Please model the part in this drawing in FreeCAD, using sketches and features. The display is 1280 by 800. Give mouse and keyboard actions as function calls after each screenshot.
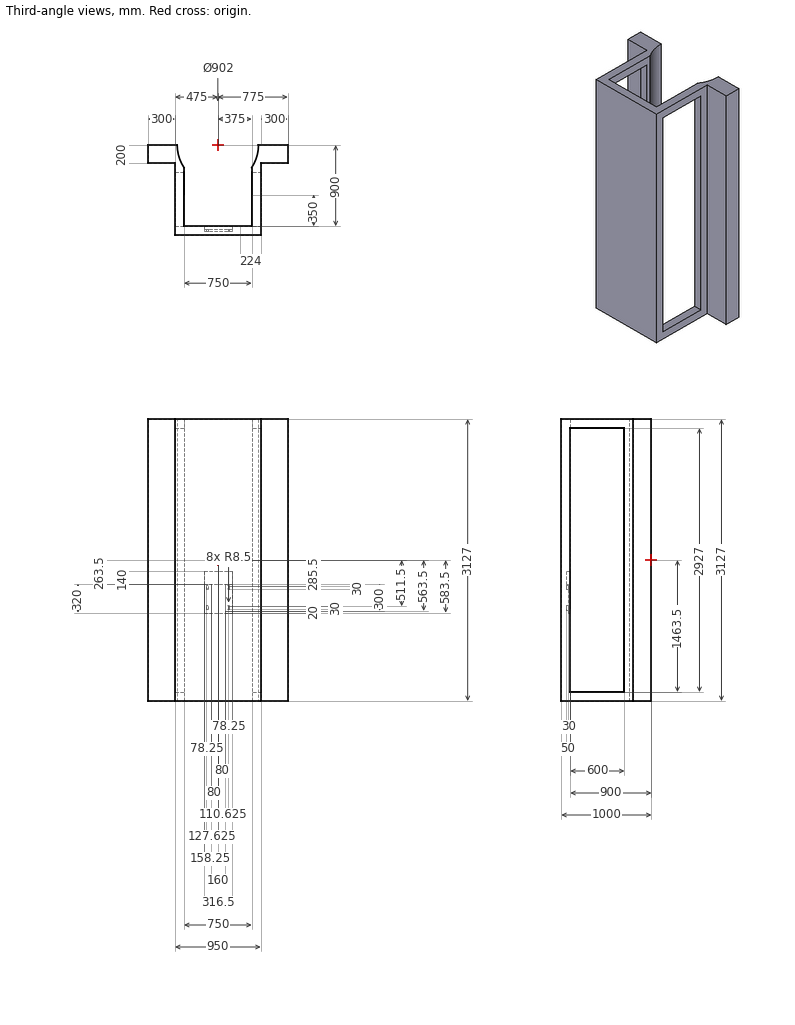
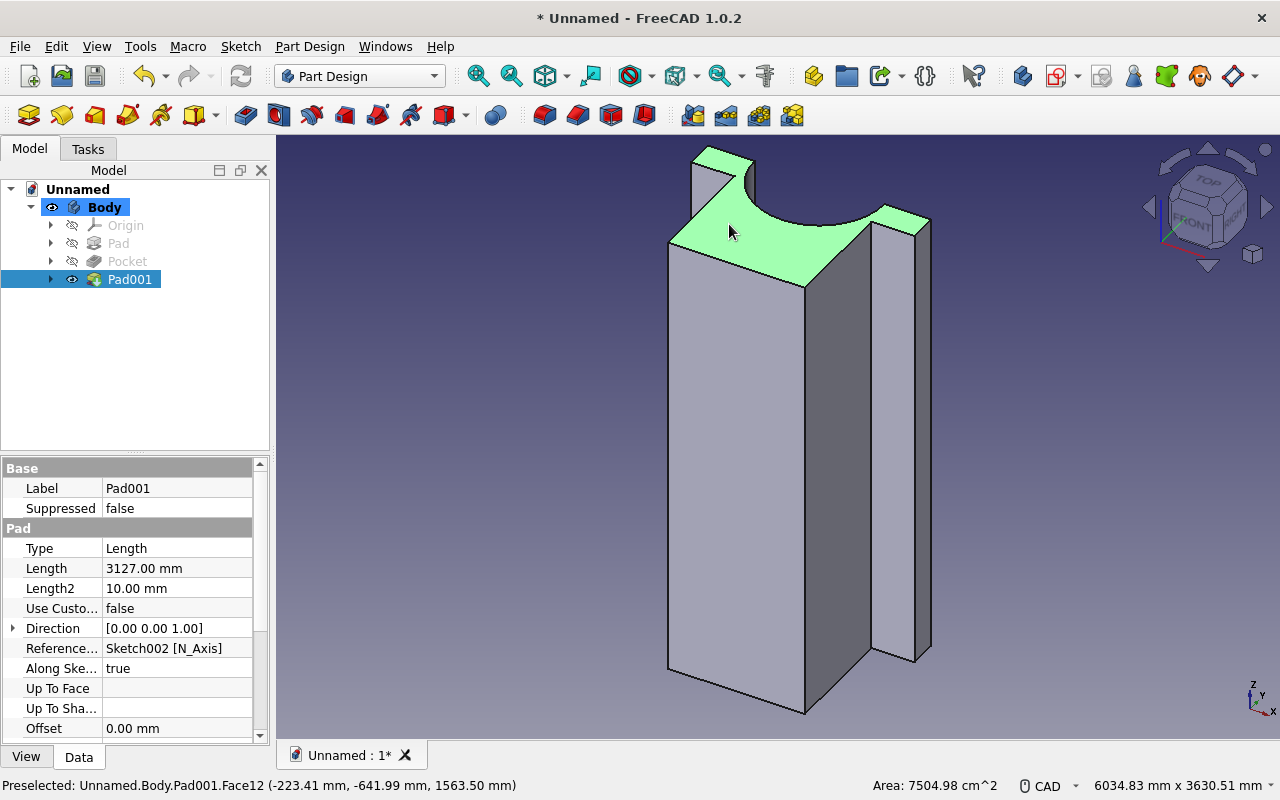
click(1056, 76)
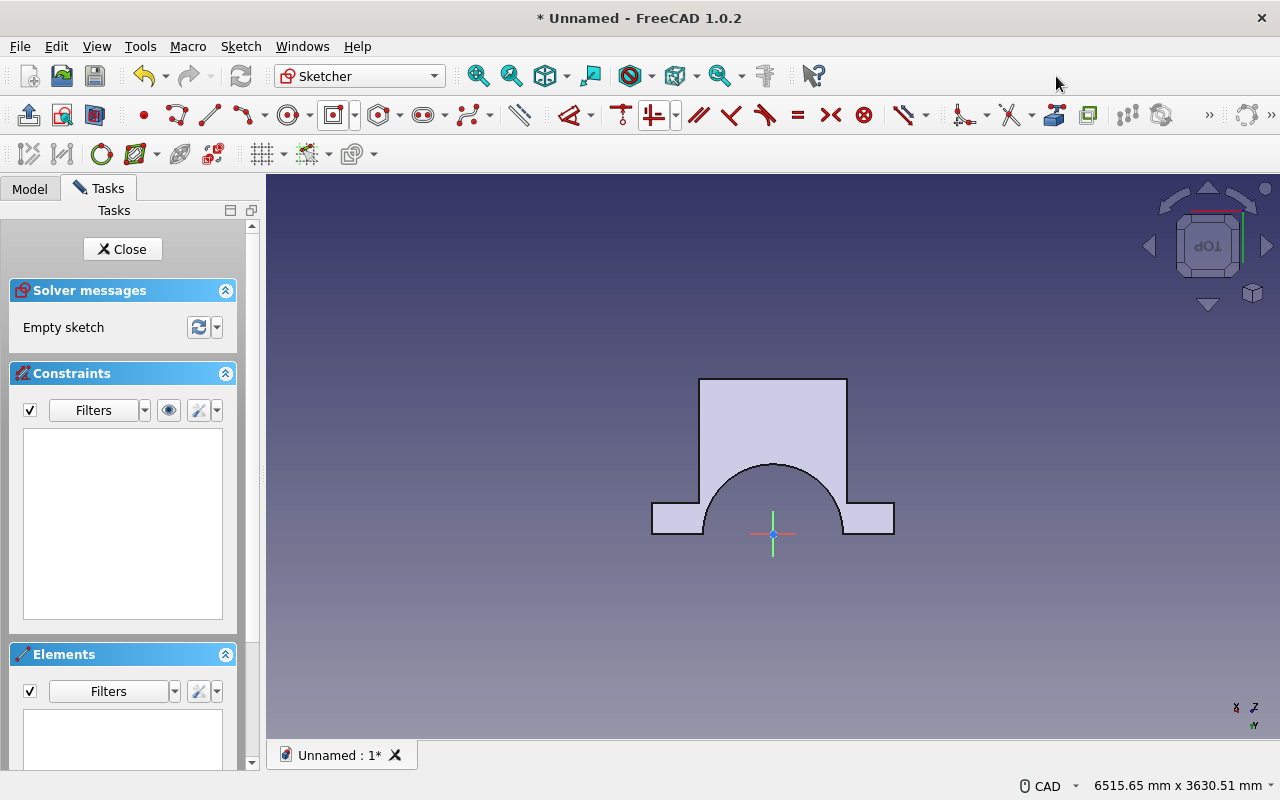
scroll(813, 469, up, 5)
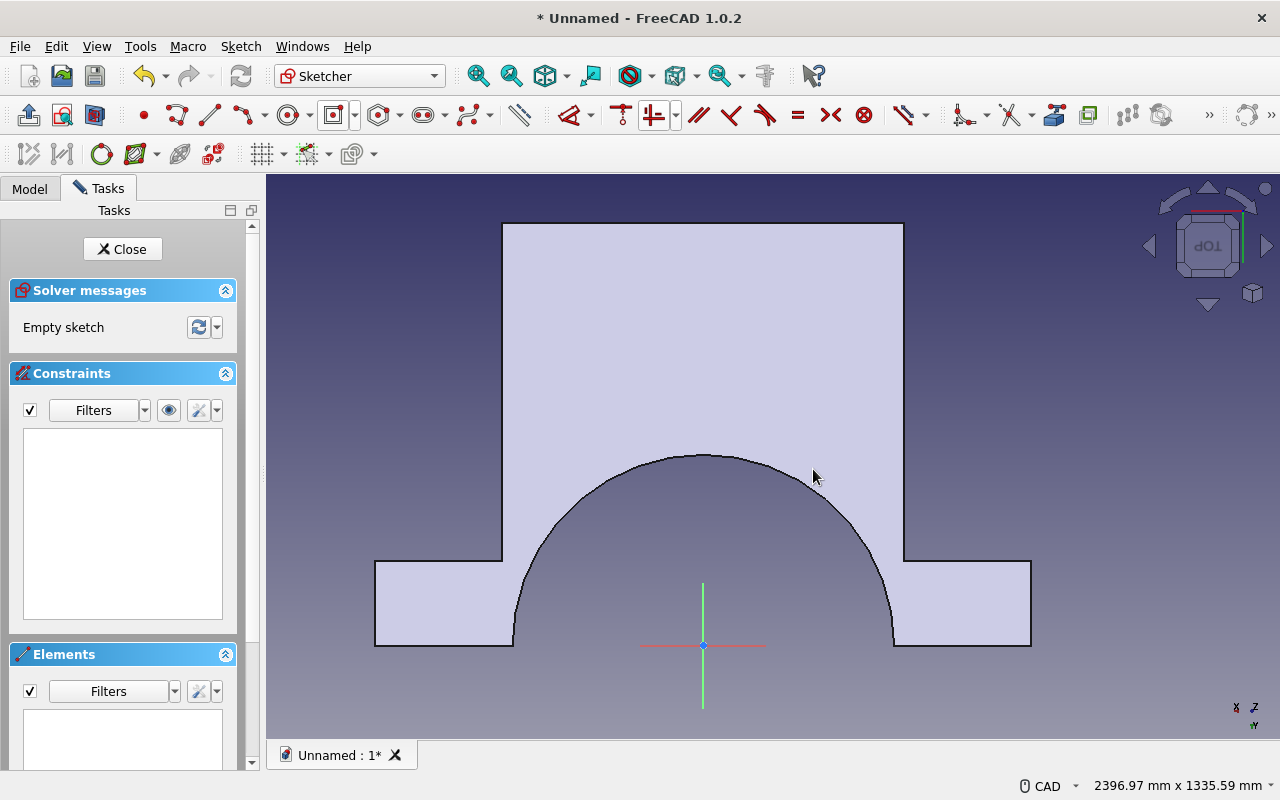
click(354, 116)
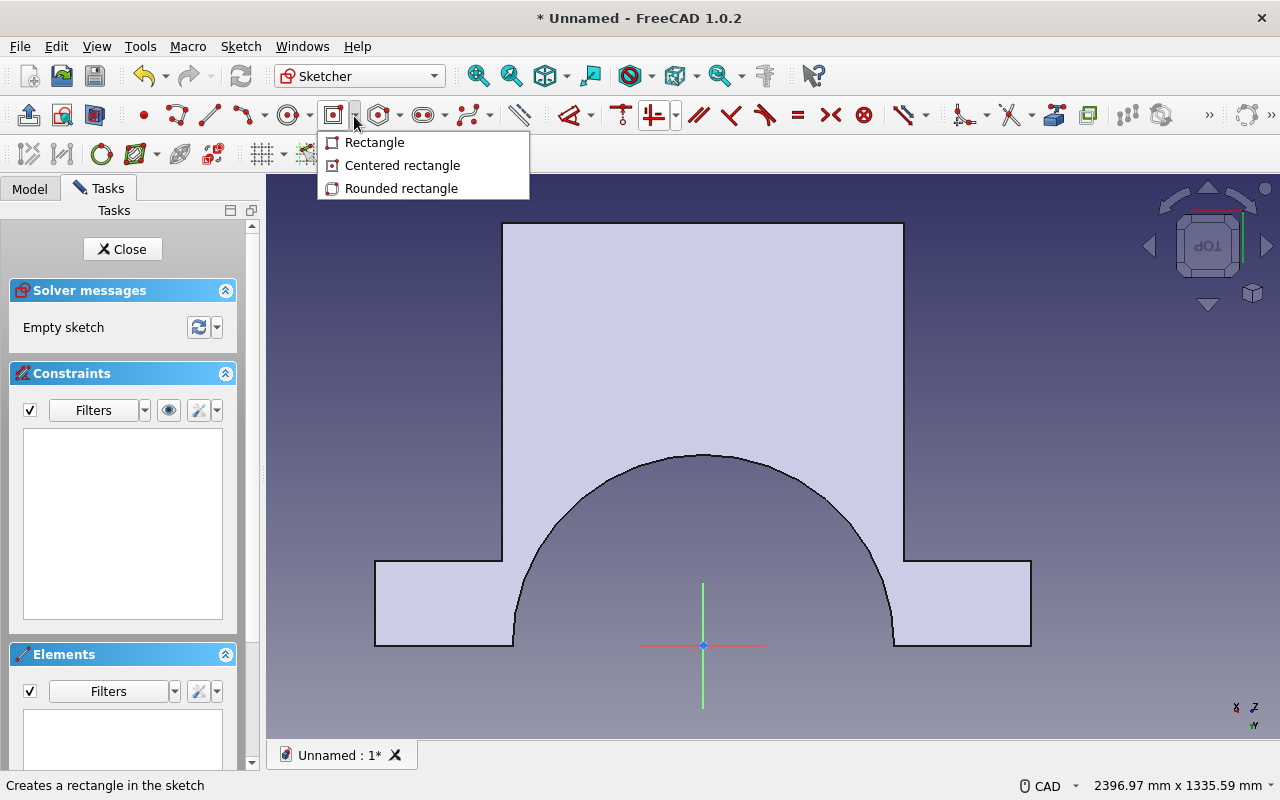
click(424, 142)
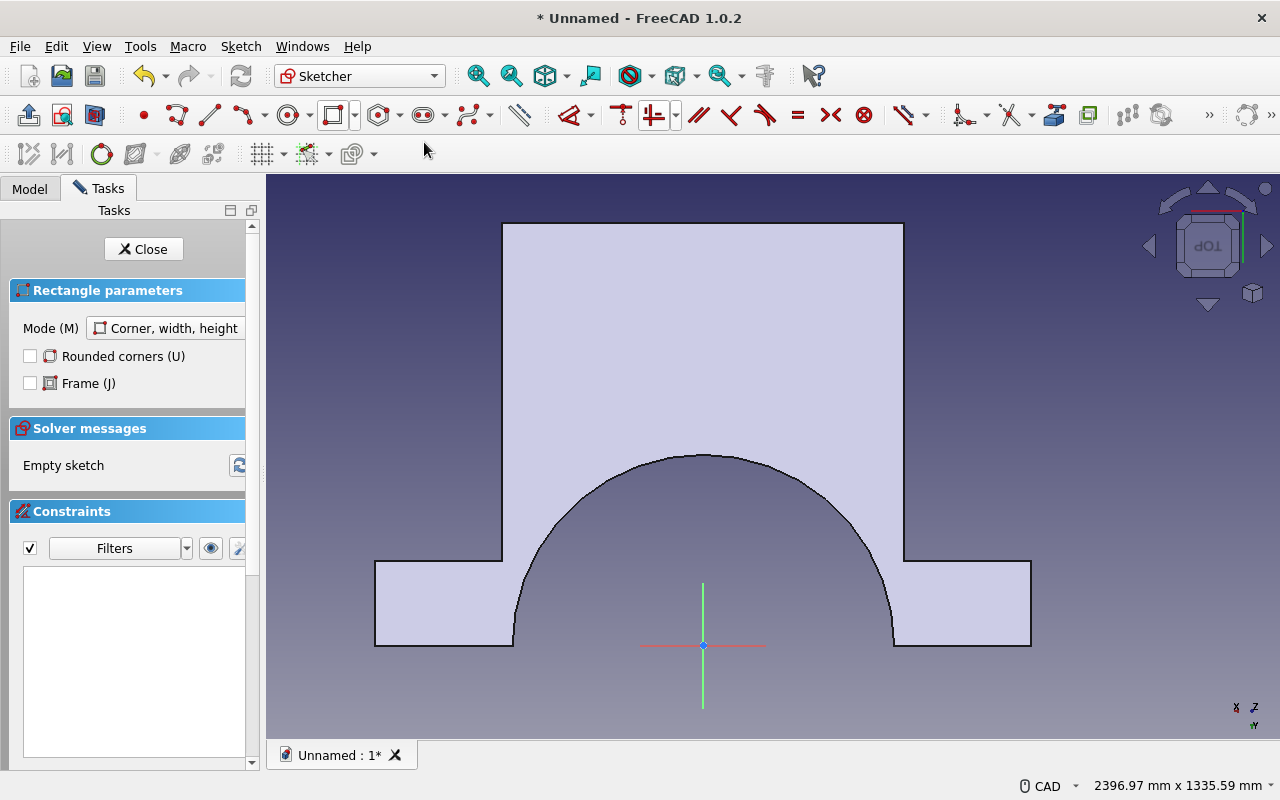
click(545, 265)
click(862, 413)
key(Escape)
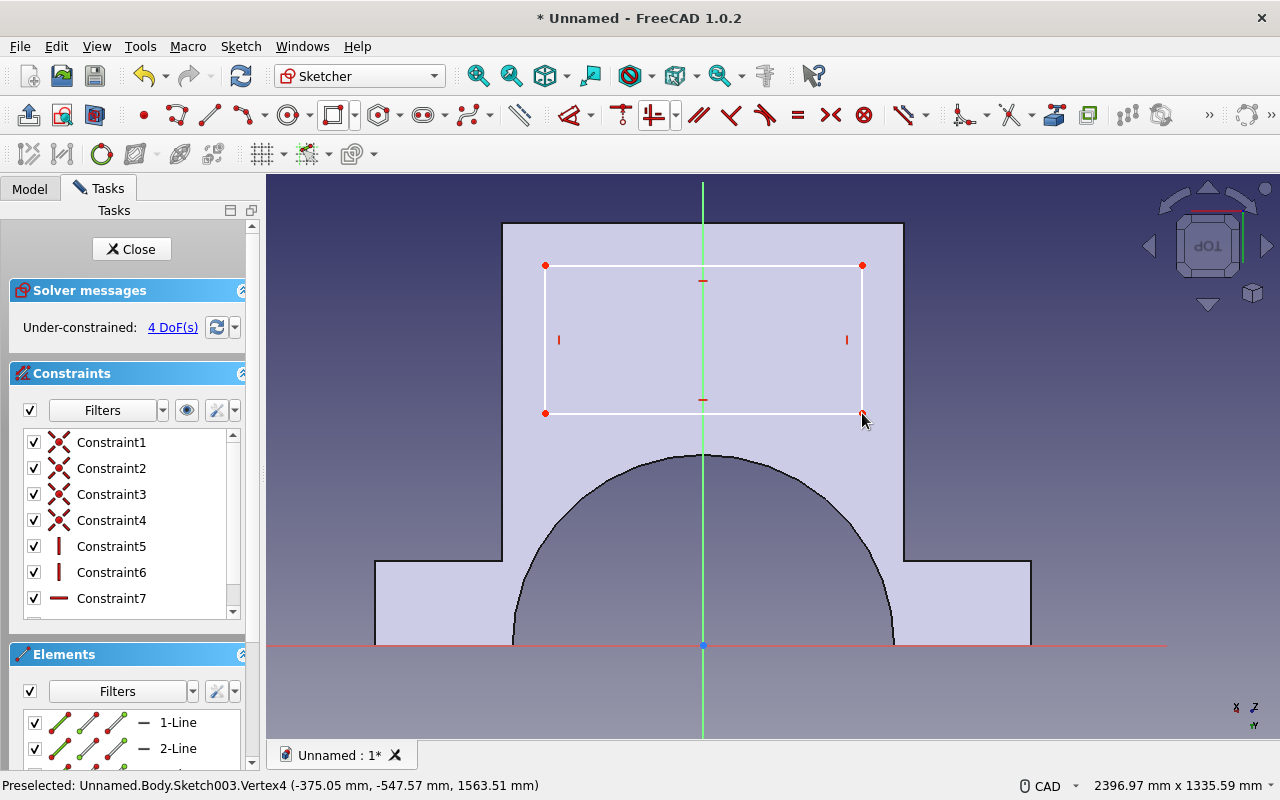
click(568, 116)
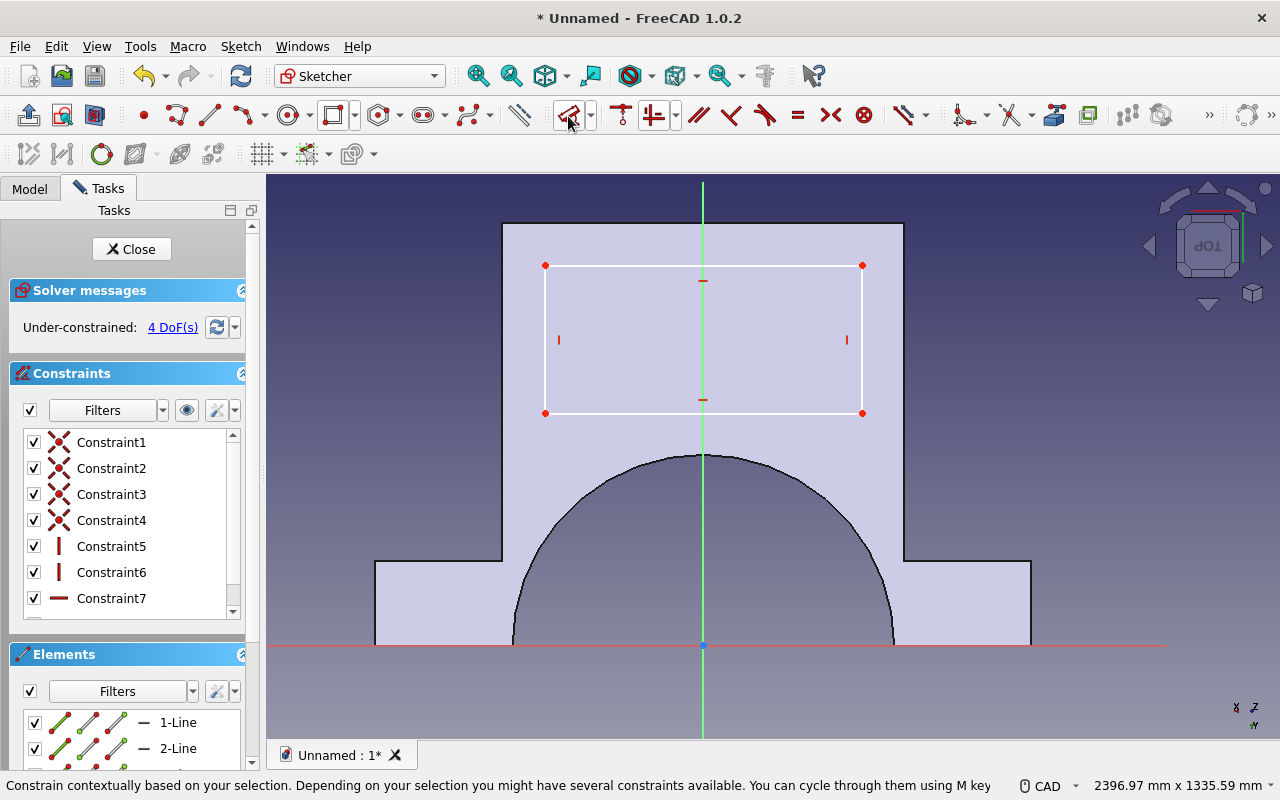
click(545, 310)
click(511, 340)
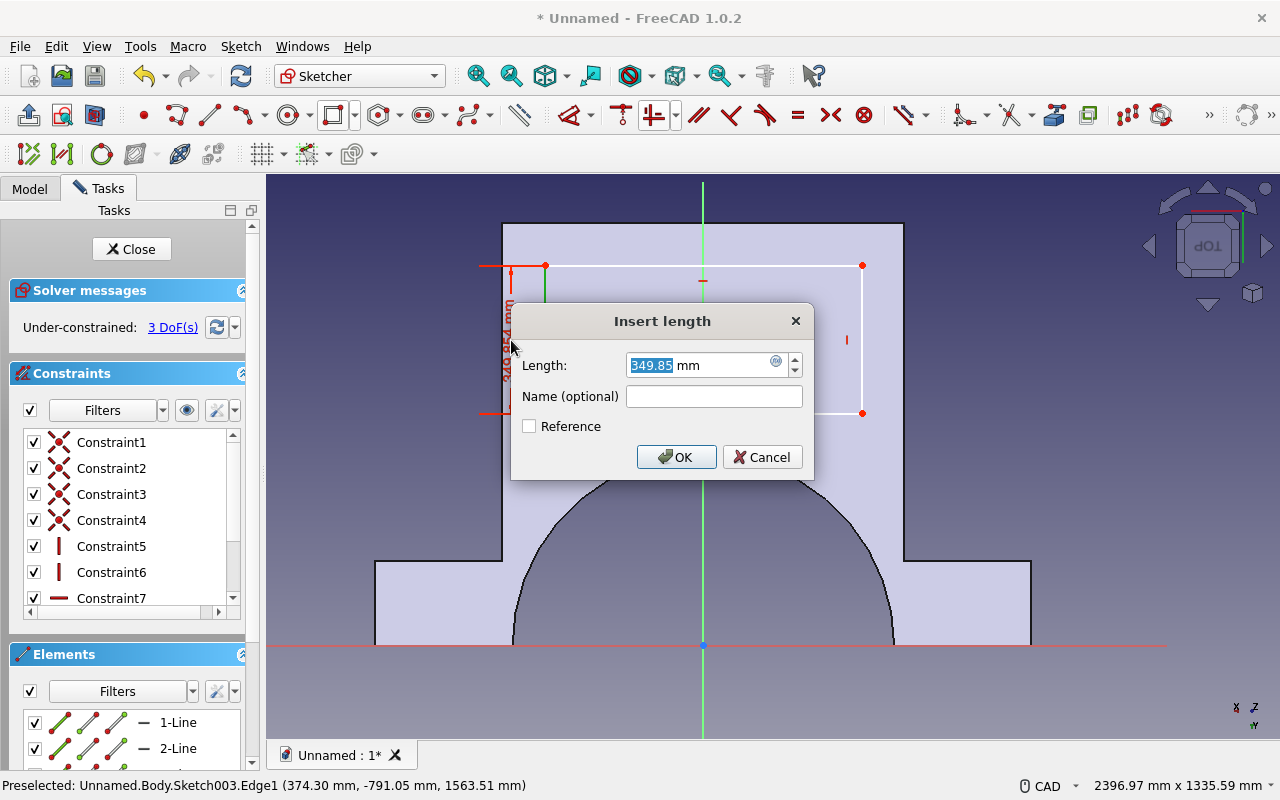
text(350)
key(Return)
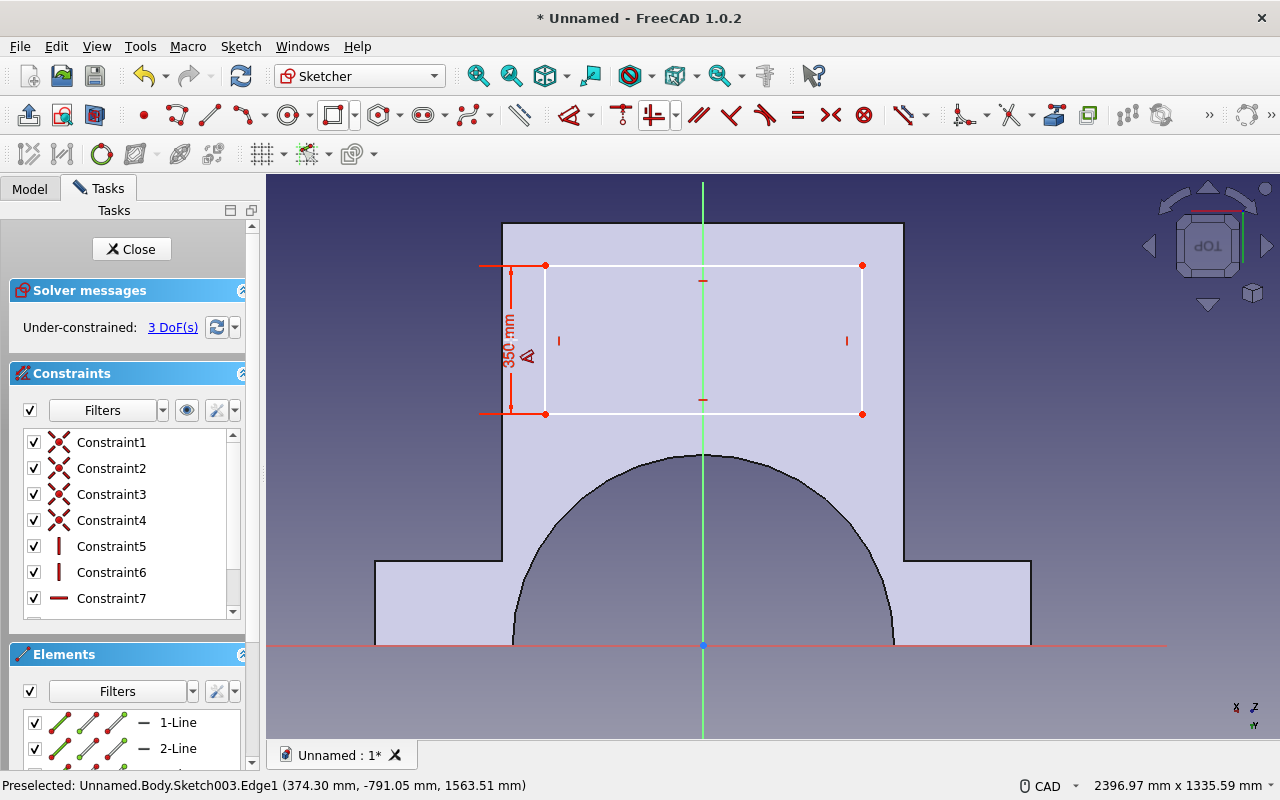
click(640, 414)
click(631, 380)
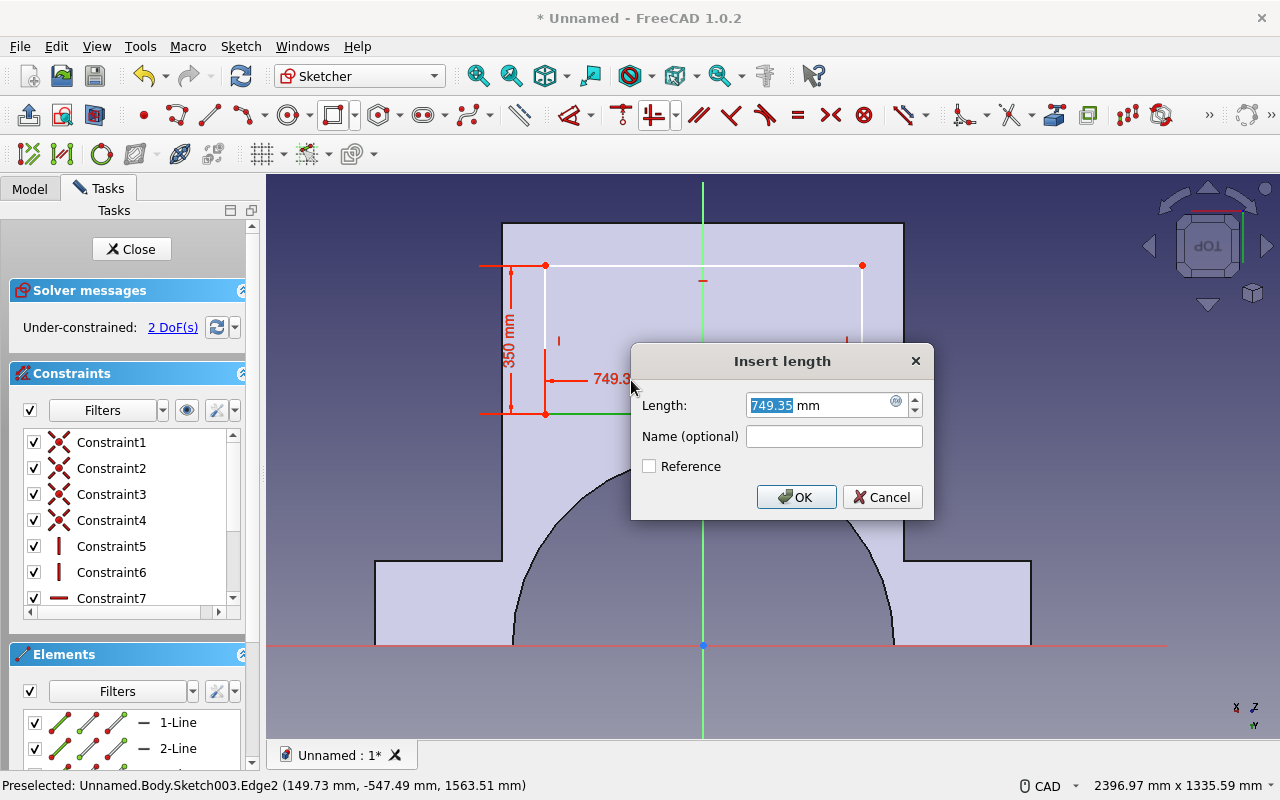
text(750)
key(Return)